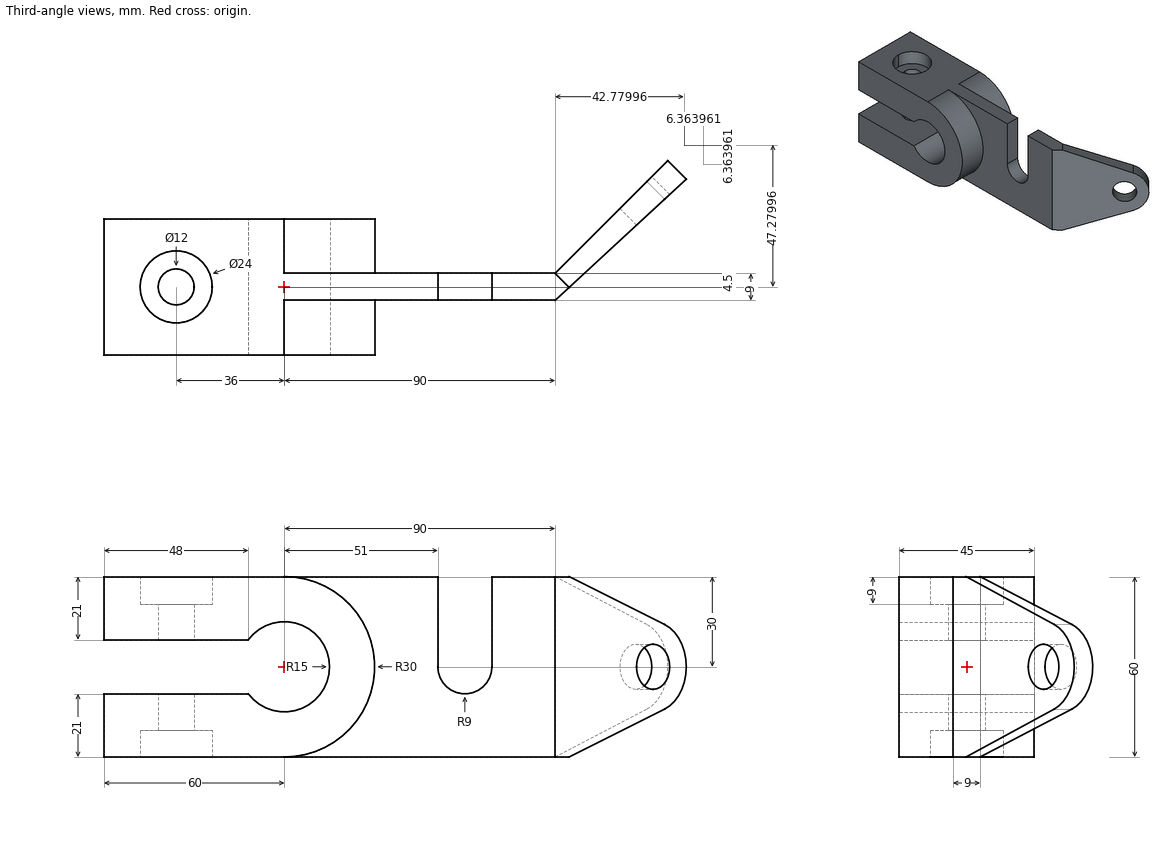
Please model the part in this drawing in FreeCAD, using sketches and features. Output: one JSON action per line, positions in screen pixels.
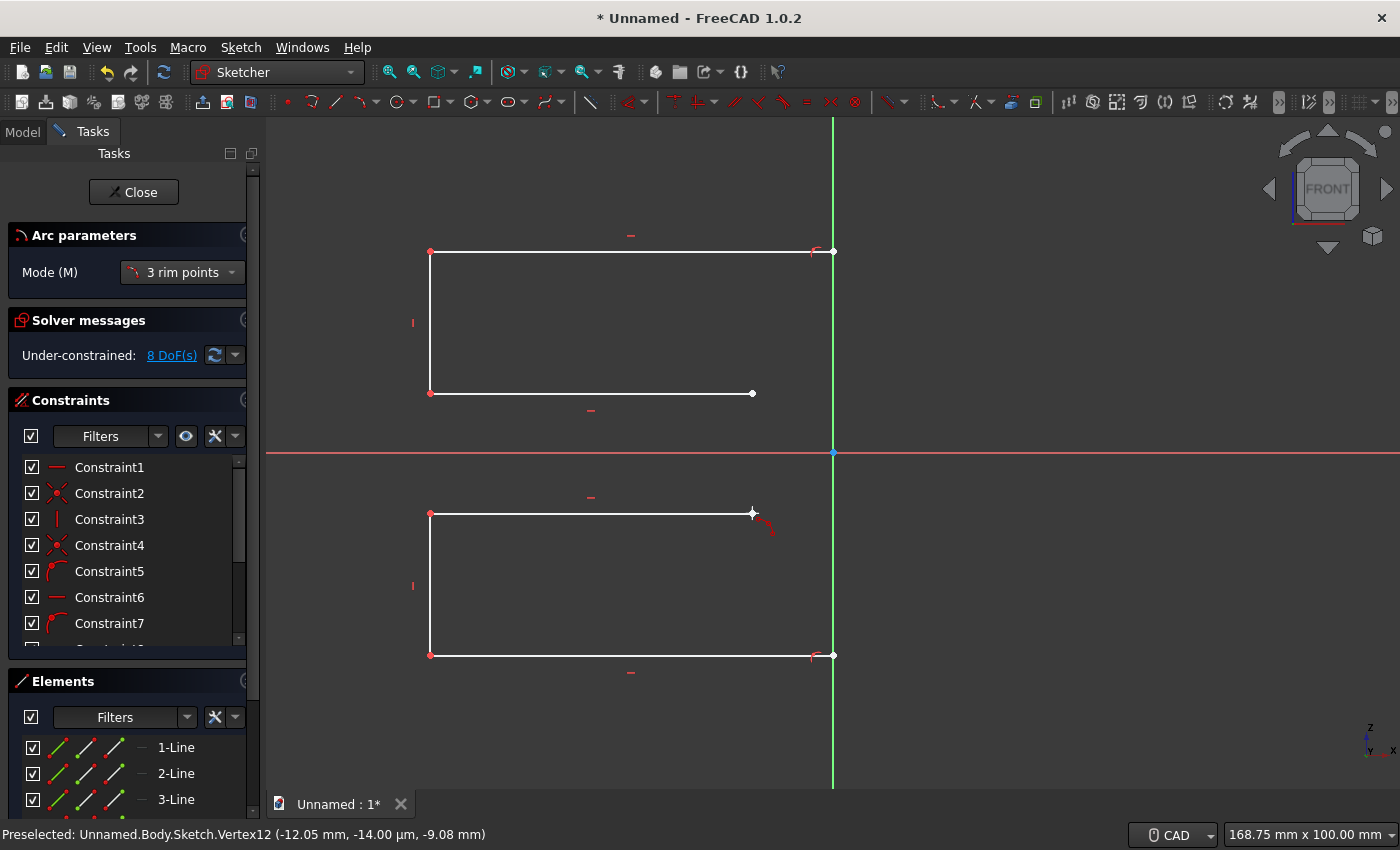
{"action": "left_click", "coordinate": [833, 252]}
{"action": "left_click", "coordinate": [833, 656]}
{"action": "left_click", "coordinate": [1025, 515]}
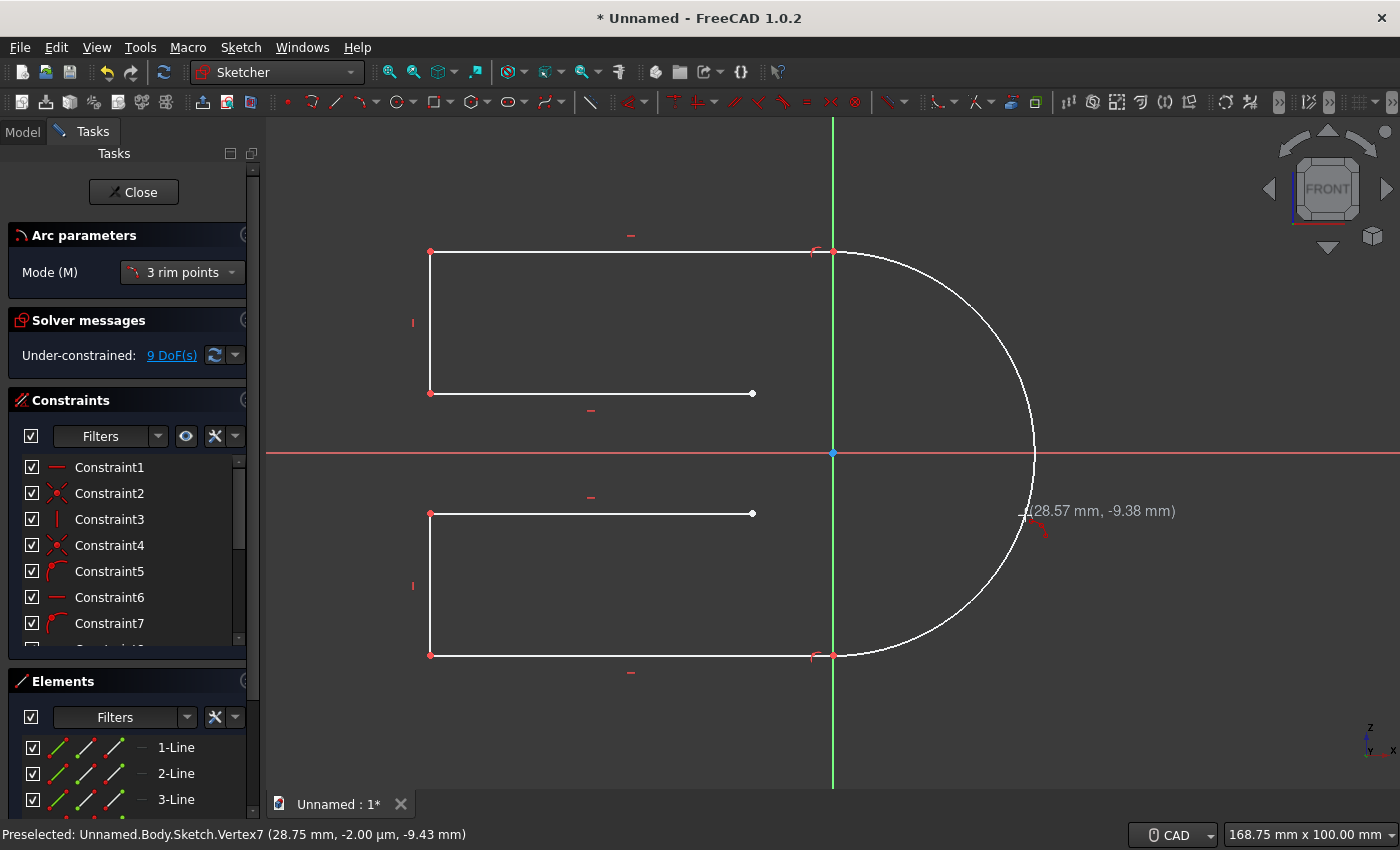
{"action": "left_click", "coordinate": [752, 514]}
{"action": "left_click", "coordinate": [752, 394]}
{"action": "left_click", "coordinate": [921, 501]}
{"action": "key", "text": "Escape"}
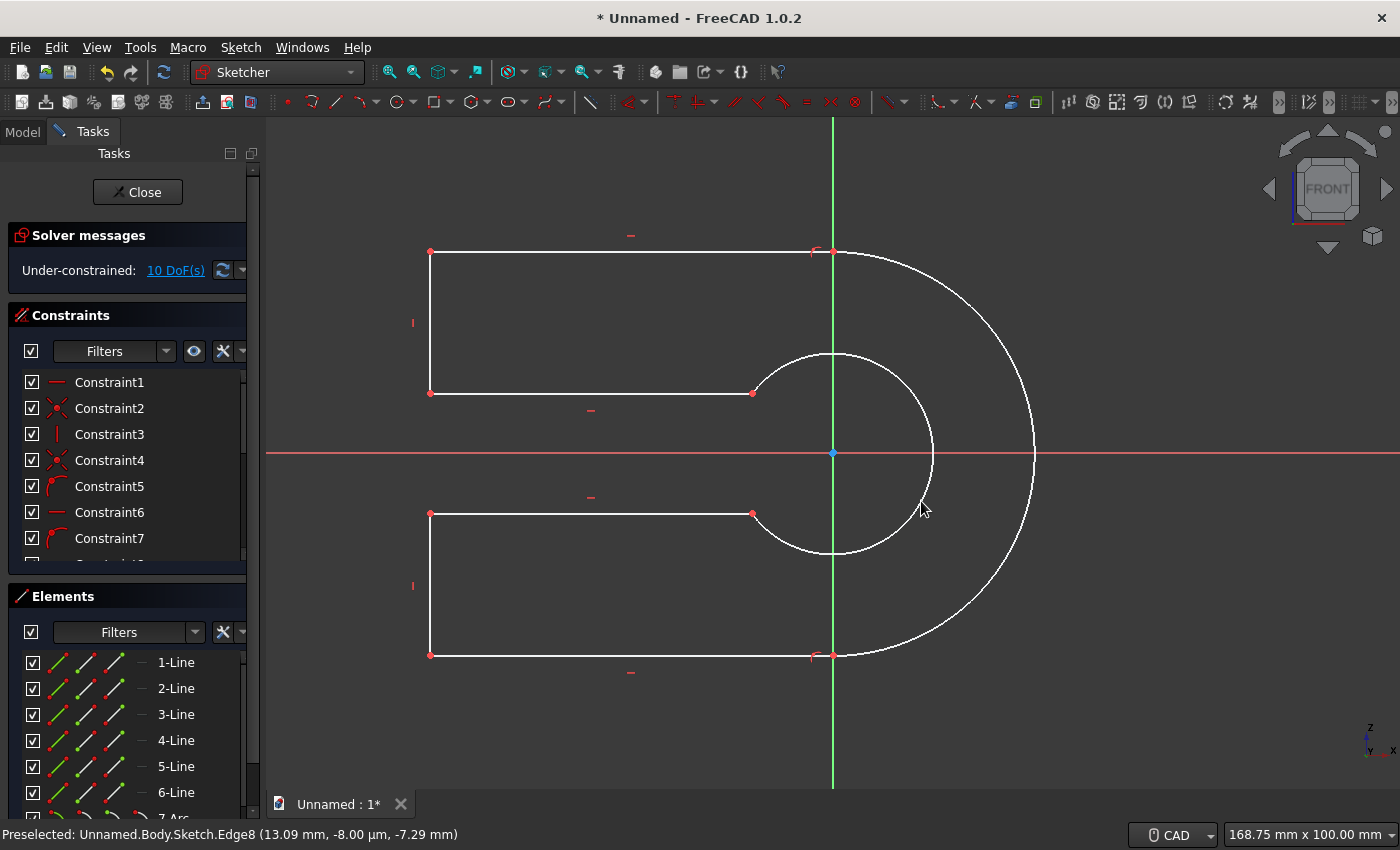
{"action": "left_click", "coordinate": [996, 573]}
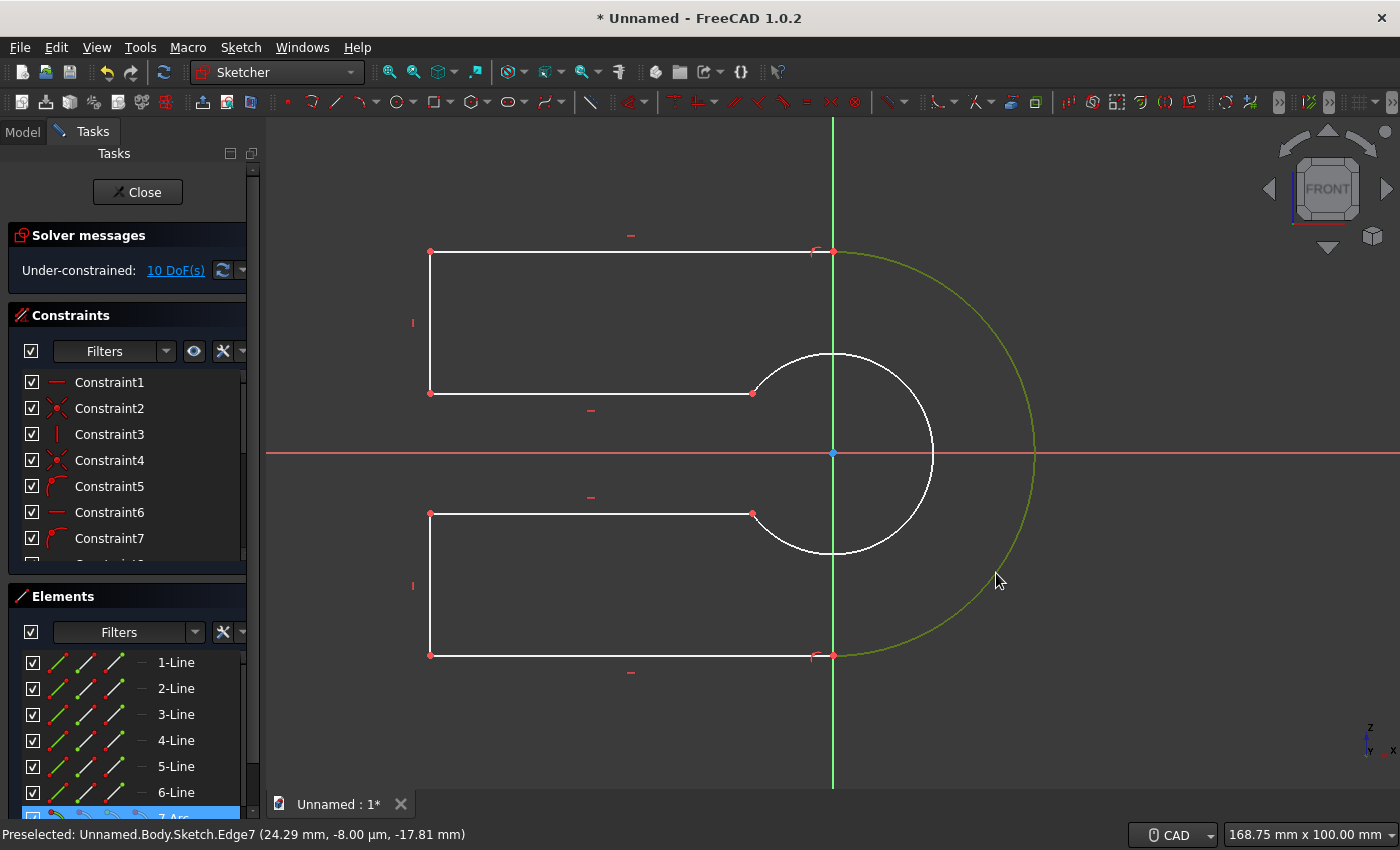
{"action": "left_click", "coordinate": [887, 539]}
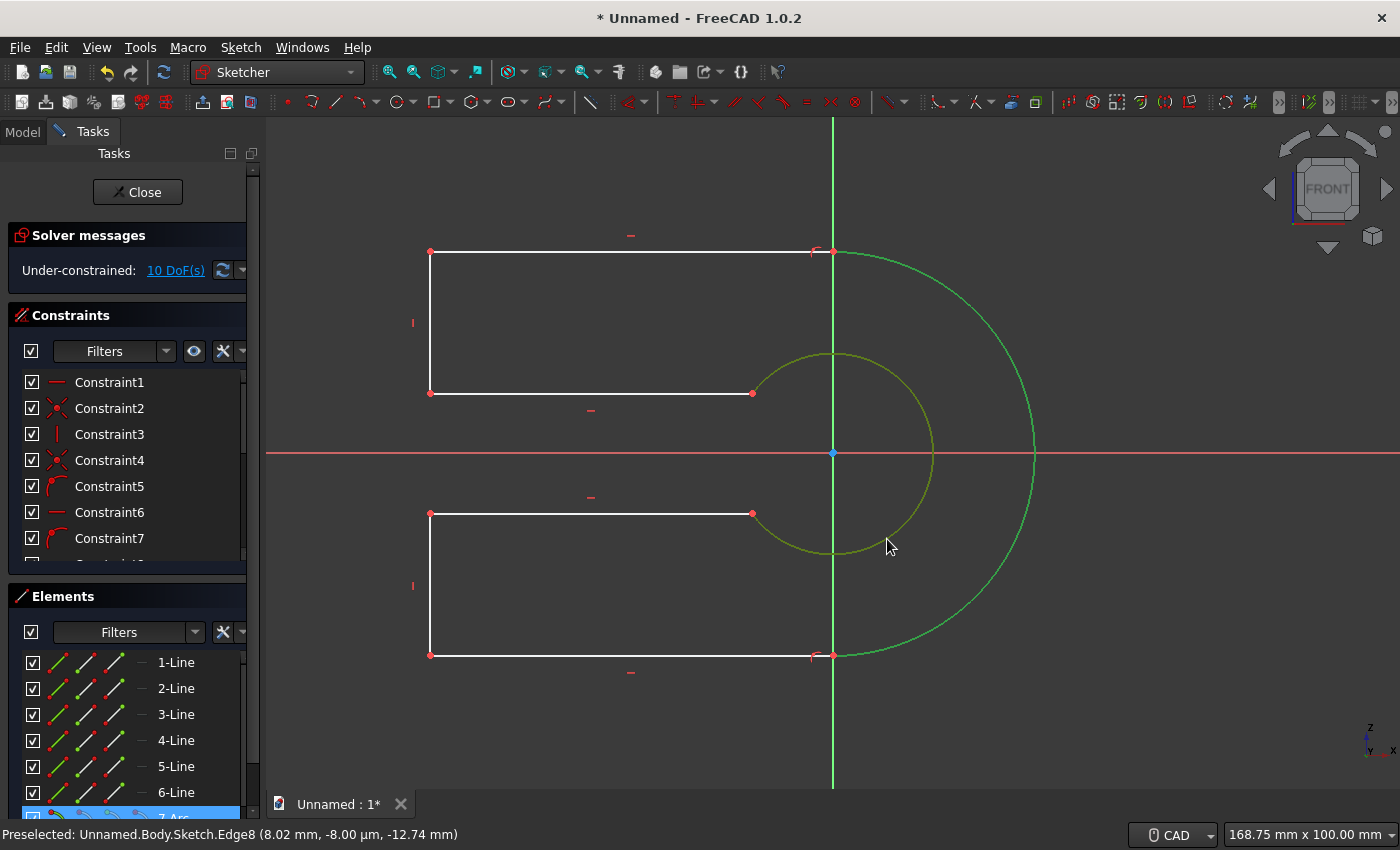
{"action": "key", "text": "c"}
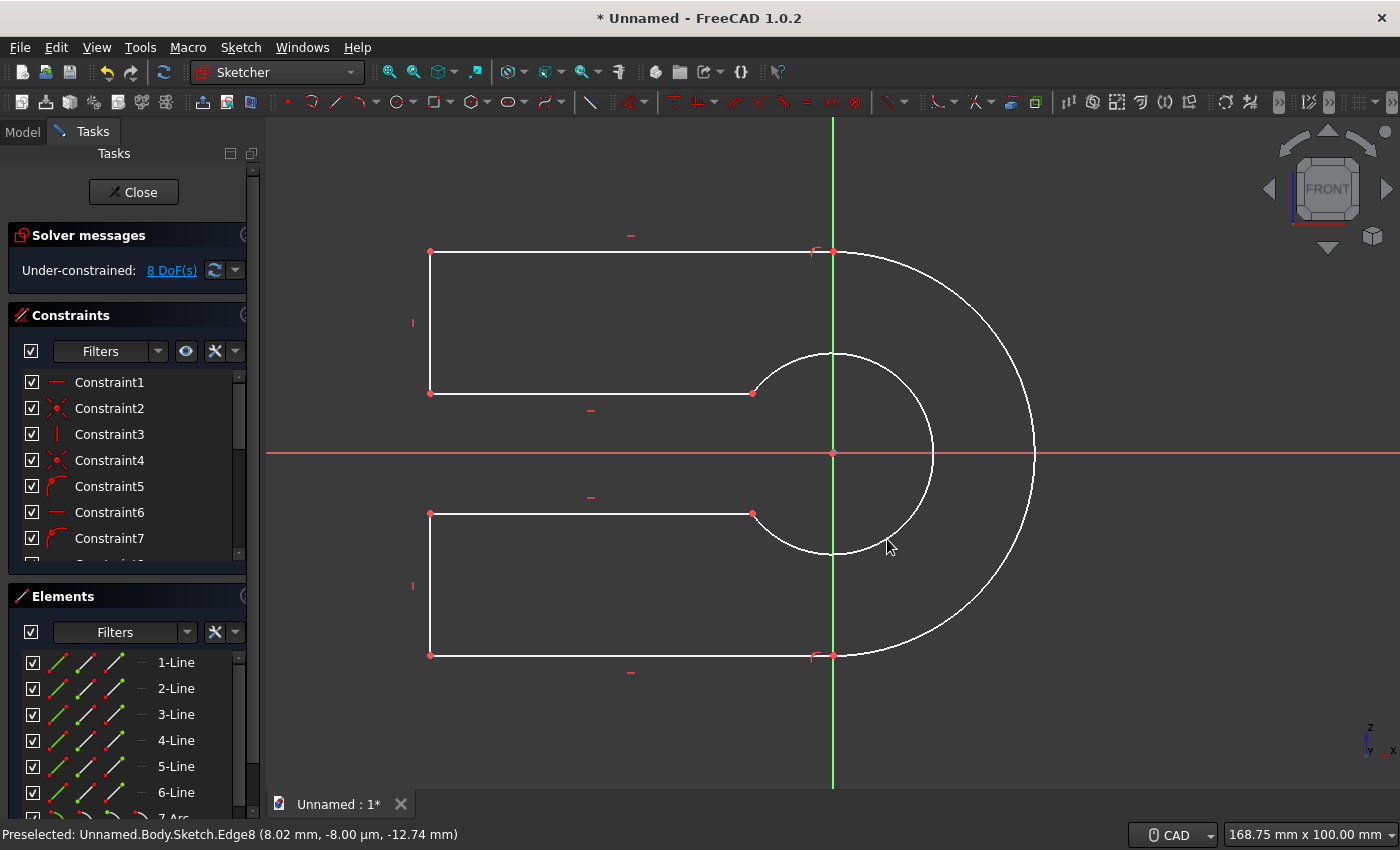
{"action": "left_click_drag", "start_coordinate": [823, 443], "coordinate": [843, 464]}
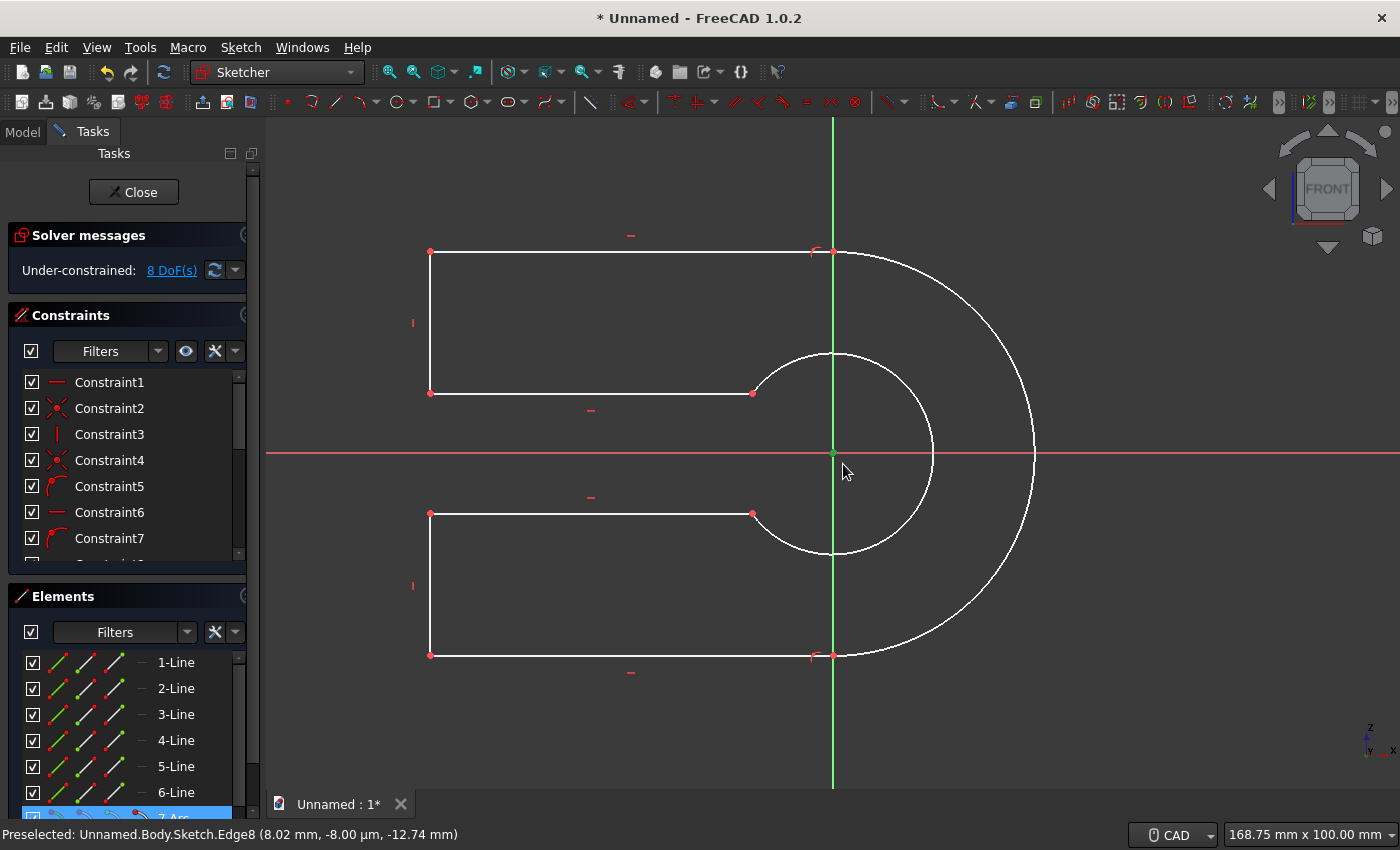
{"action": "key", "text": "c"}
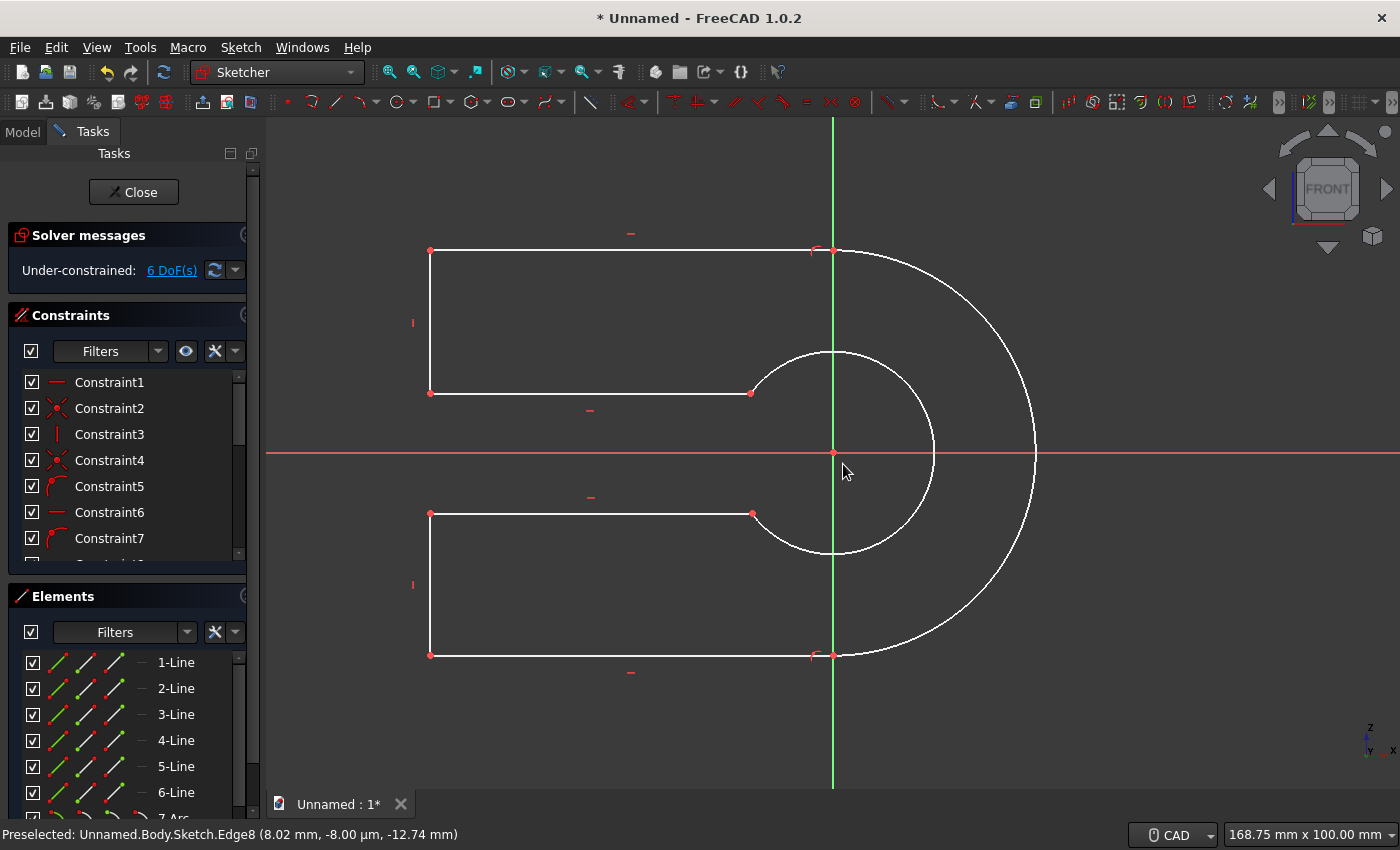
{"action": "left_click", "coordinate": [628, 102]}